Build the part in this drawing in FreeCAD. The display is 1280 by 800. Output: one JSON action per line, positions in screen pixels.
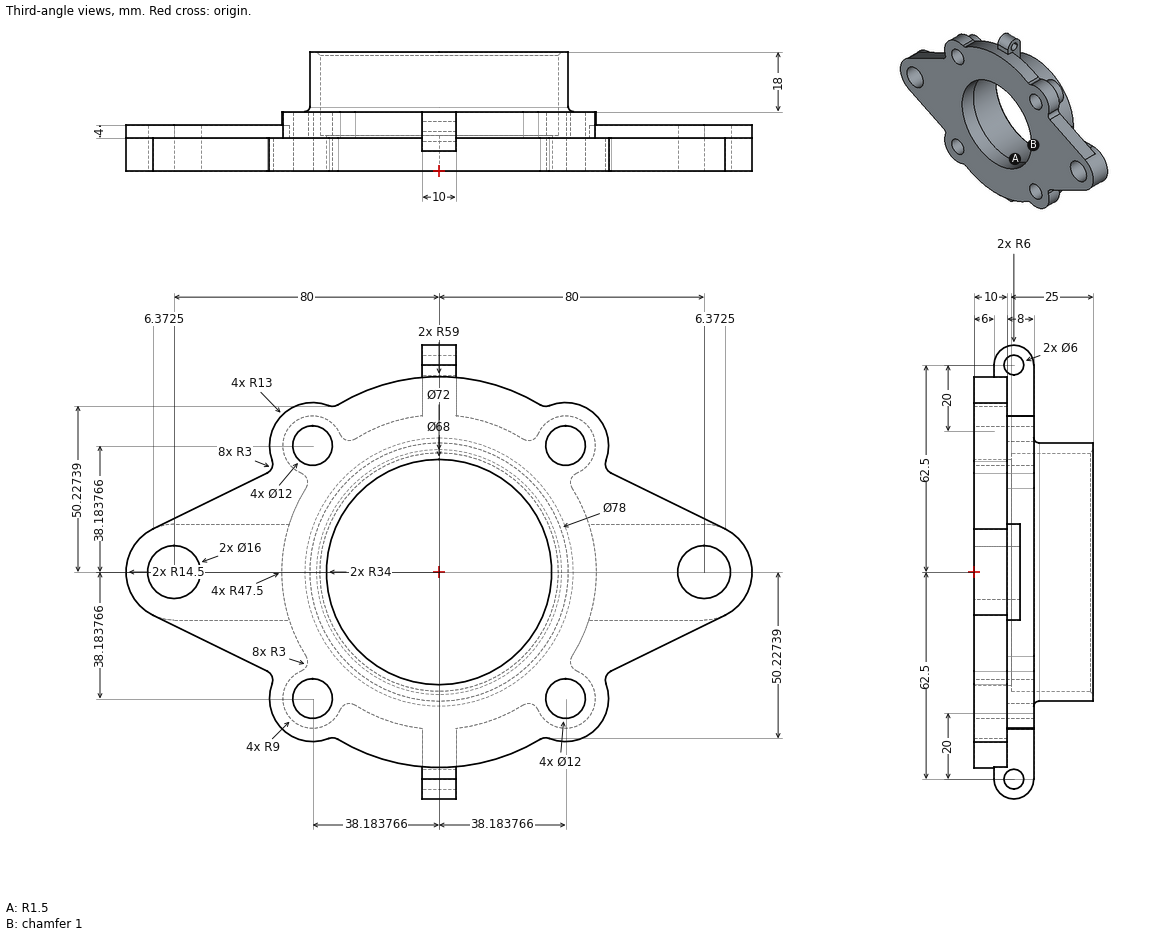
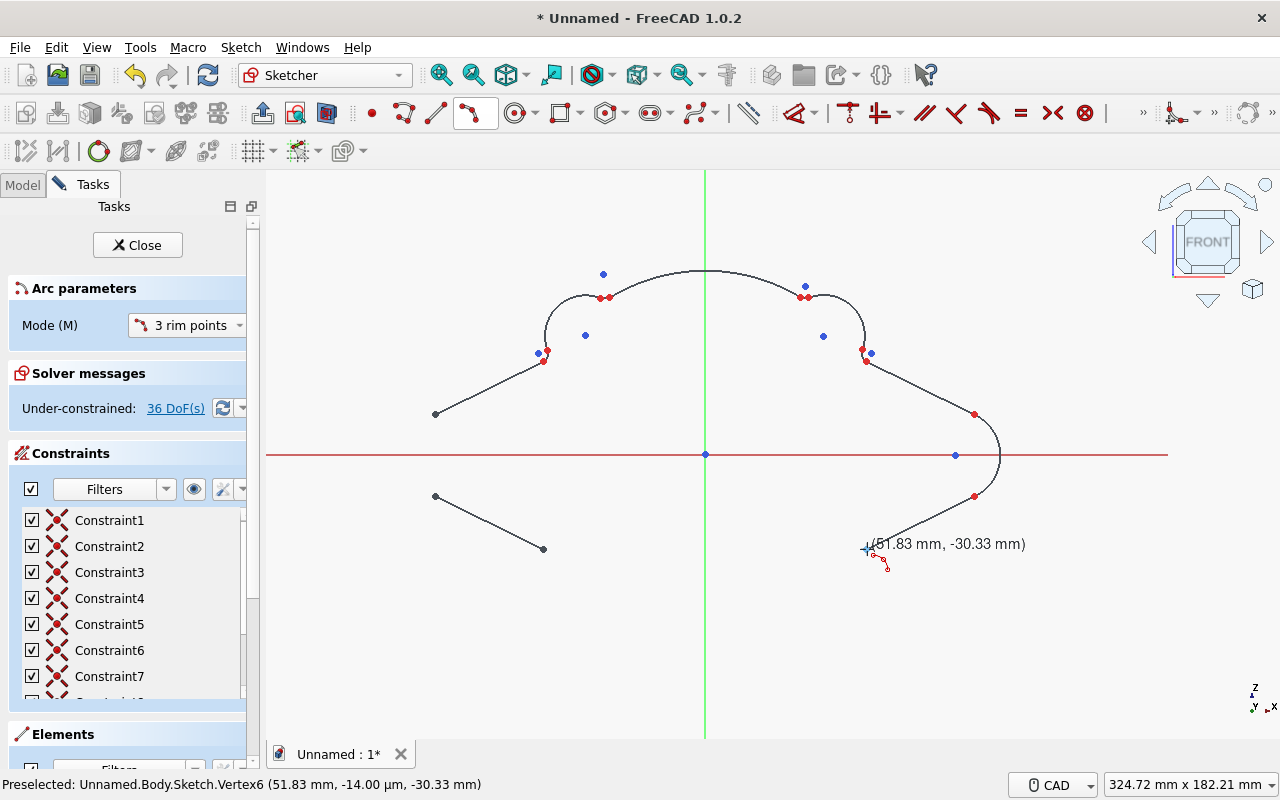
{"action": "scroll", "coordinate": [862, 560], "scroll_direction": "up", "scroll_amount": 2}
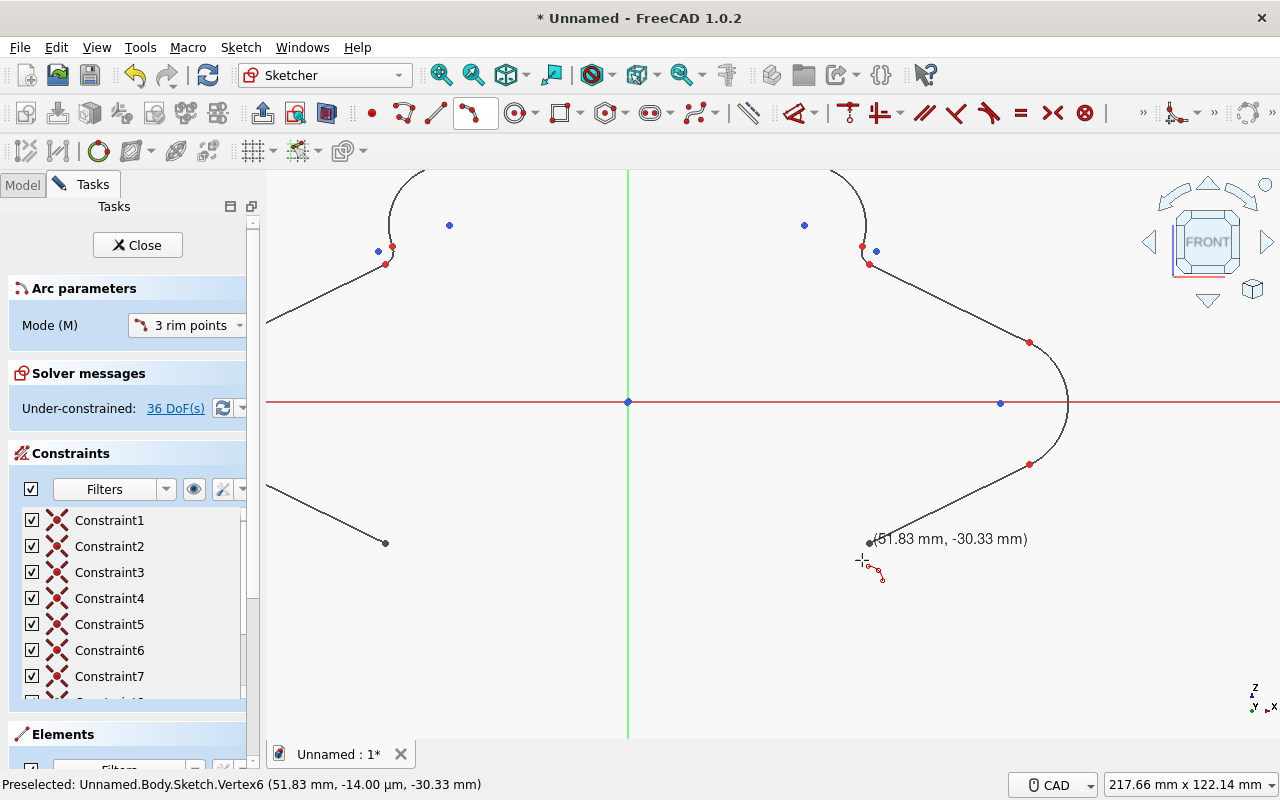
{"action": "left_click", "coordinate": [862, 559]}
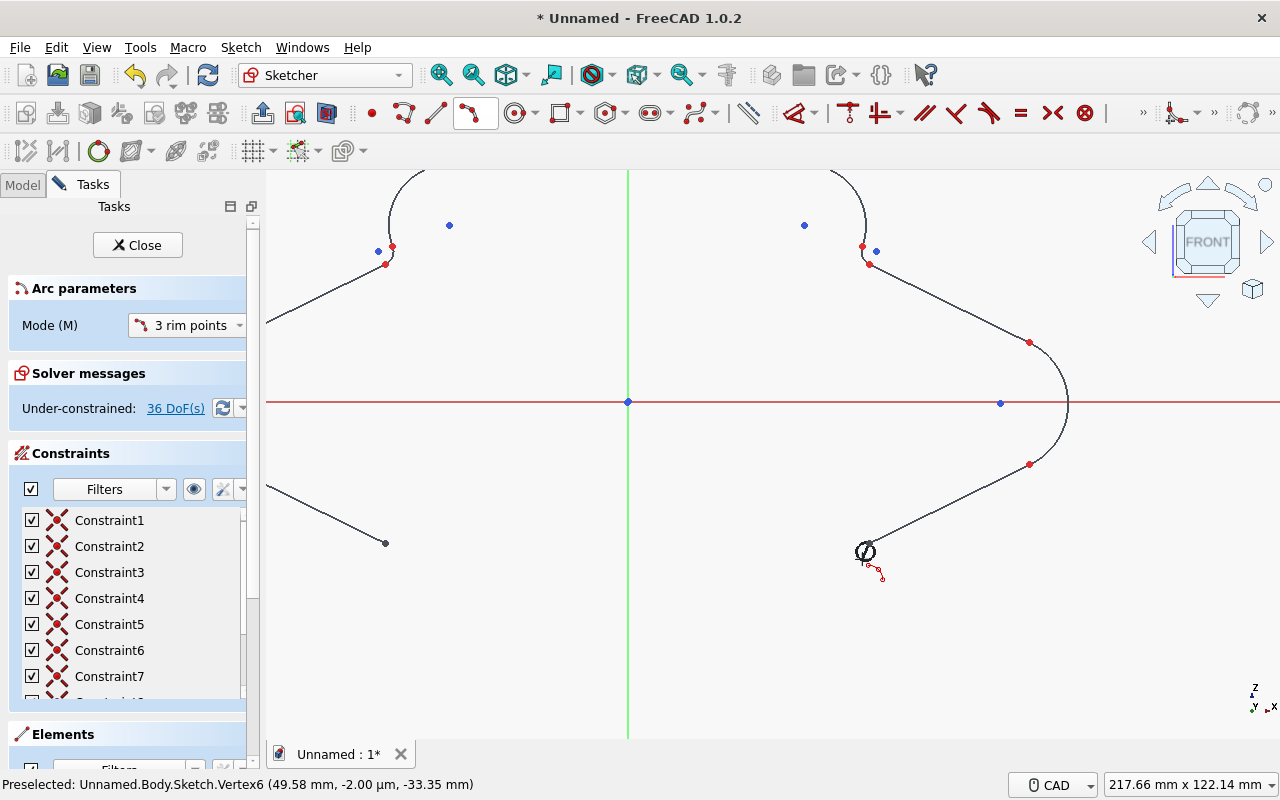
{"action": "scroll", "coordinate": [862, 549], "scroll_direction": "up", "scroll_amount": 8}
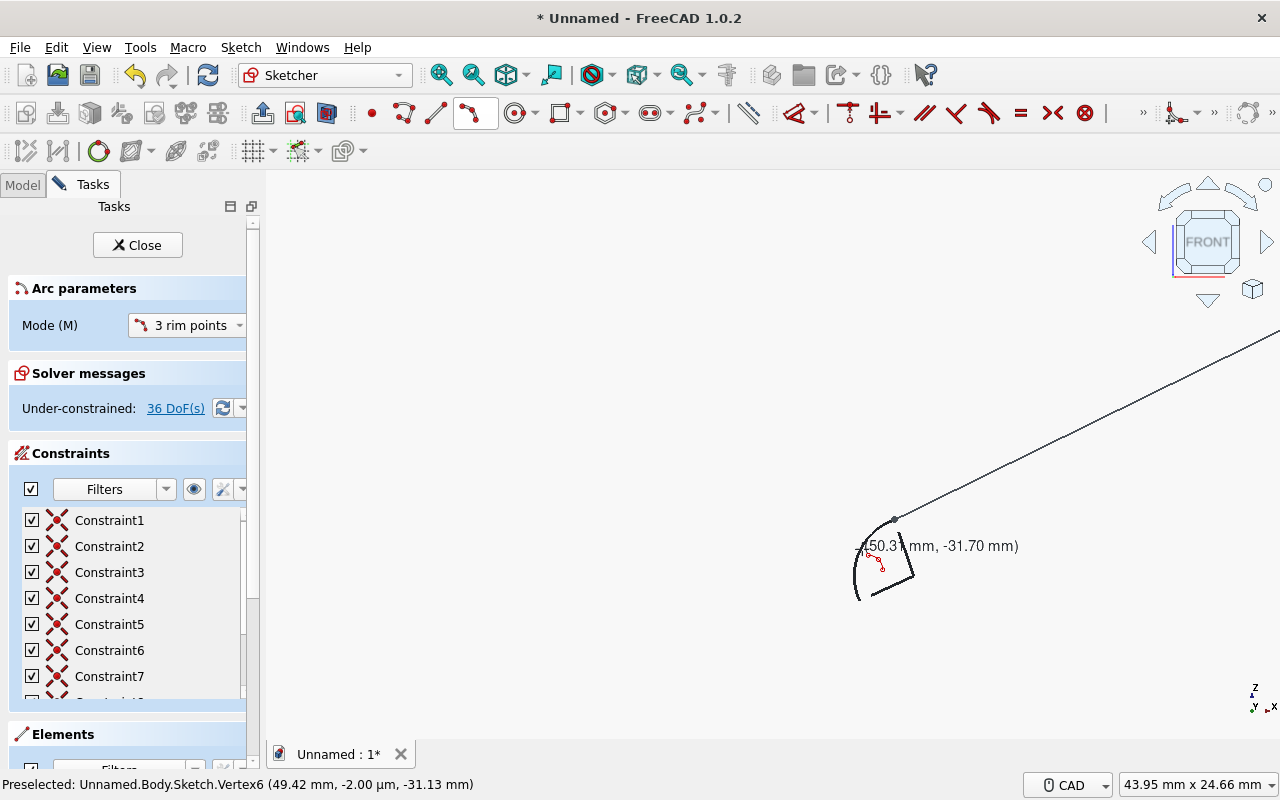
{"action": "left_click", "coordinate": [862, 547]}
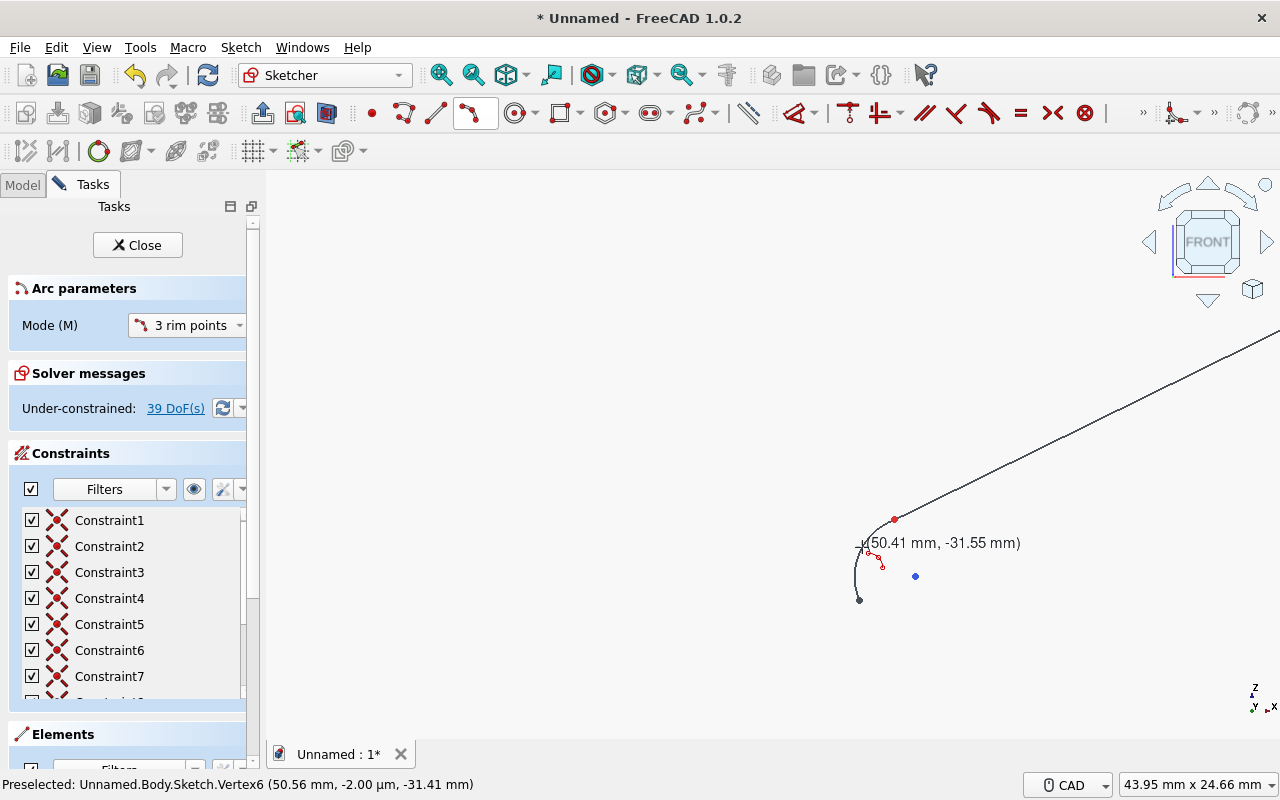
{"action": "scroll", "coordinate": [862, 554], "scroll_direction": "down", "scroll_amount": 10}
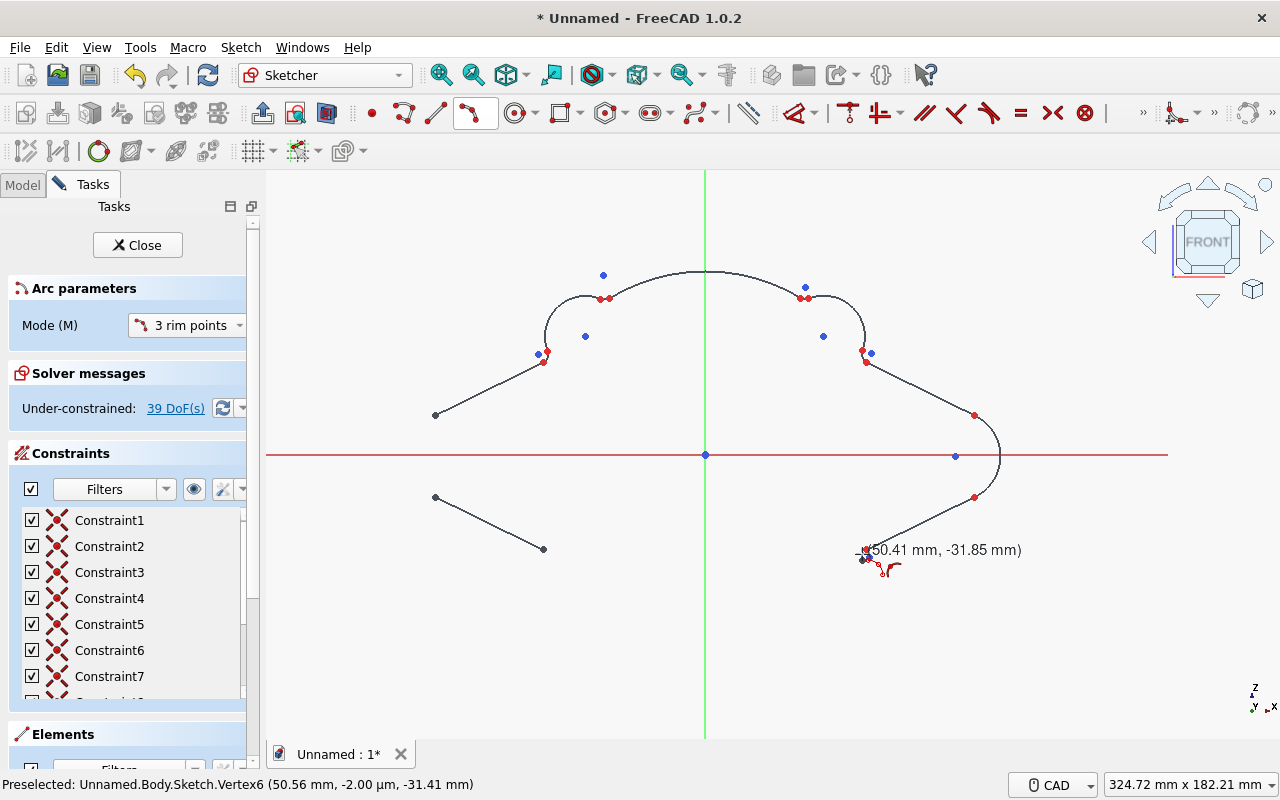
{"action": "scroll", "coordinate": [862, 560], "scroll_direction": "up", "scroll_amount": 3}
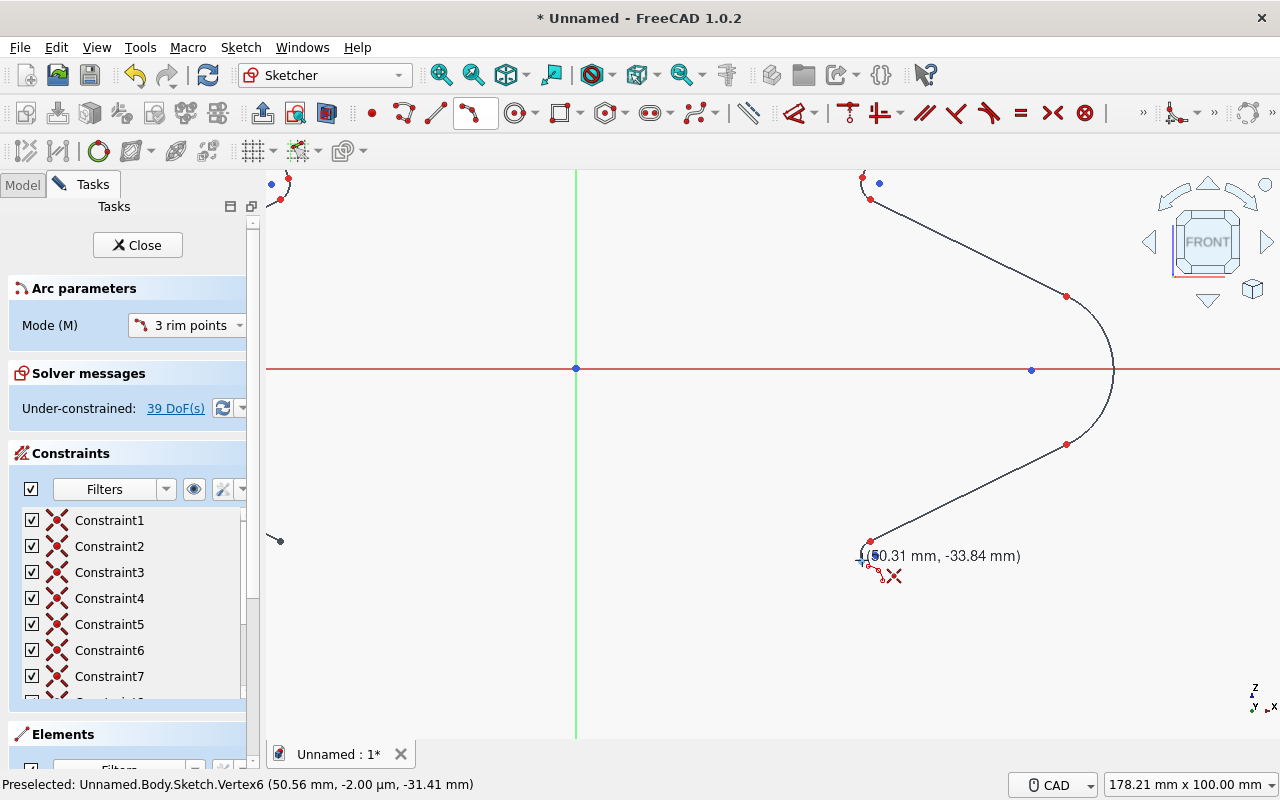
{"action": "left_click", "coordinate": [862, 561]}
{"action": "left_click", "coordinate": [765, 654]}
{"action": "left_click", "coordinate": [844, 639]}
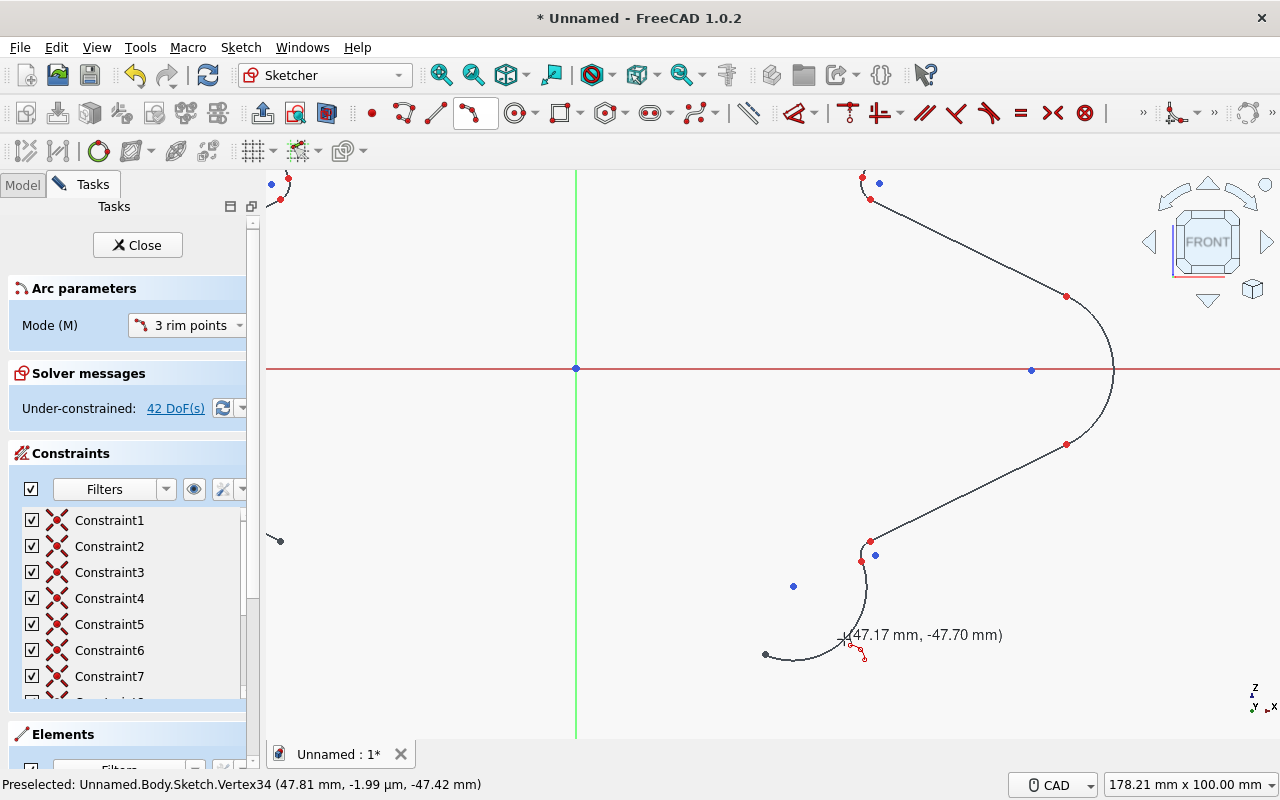
{"action": "left_click", "coordinate": [765, 655]}
{"action": "left_click", "coordinate": [750, 656]}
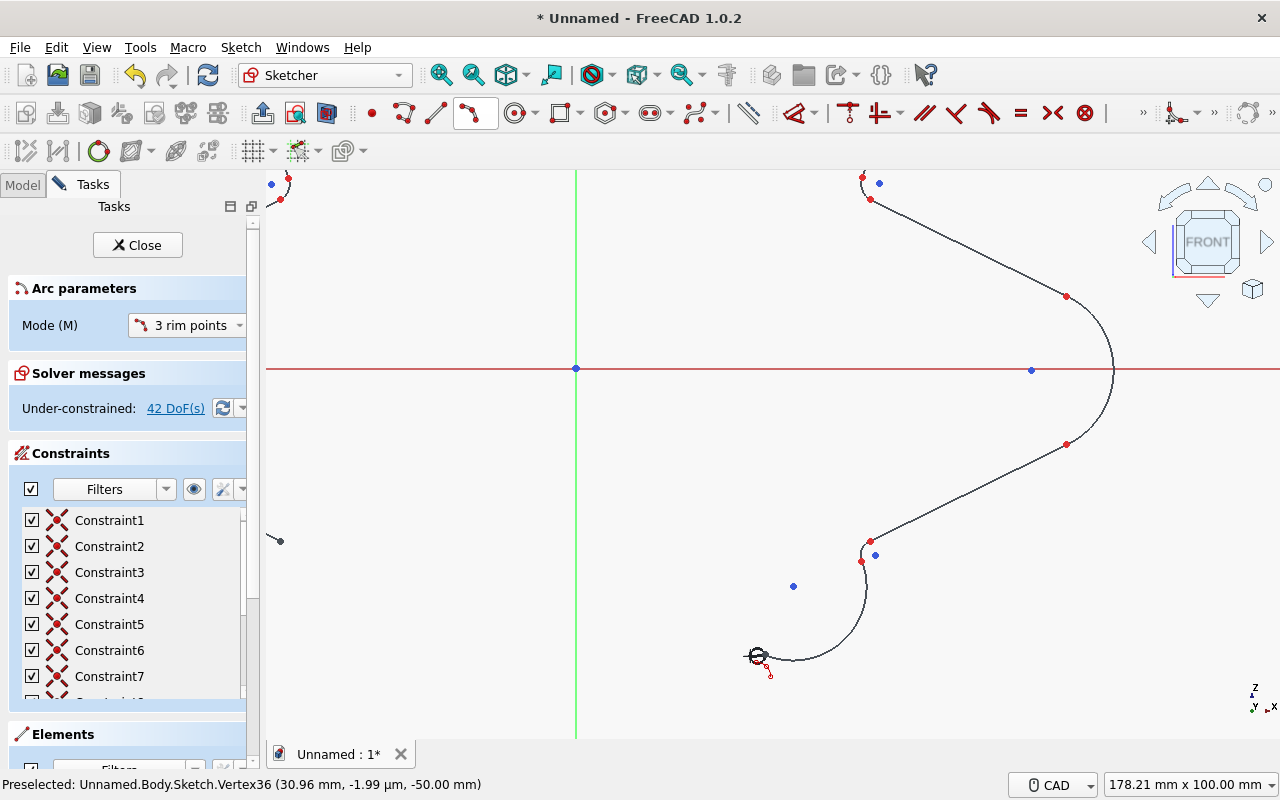
{"action": "scroll", "coordinate": [757, 653], "scroll_direction": "up", "scroll_amount": 11}